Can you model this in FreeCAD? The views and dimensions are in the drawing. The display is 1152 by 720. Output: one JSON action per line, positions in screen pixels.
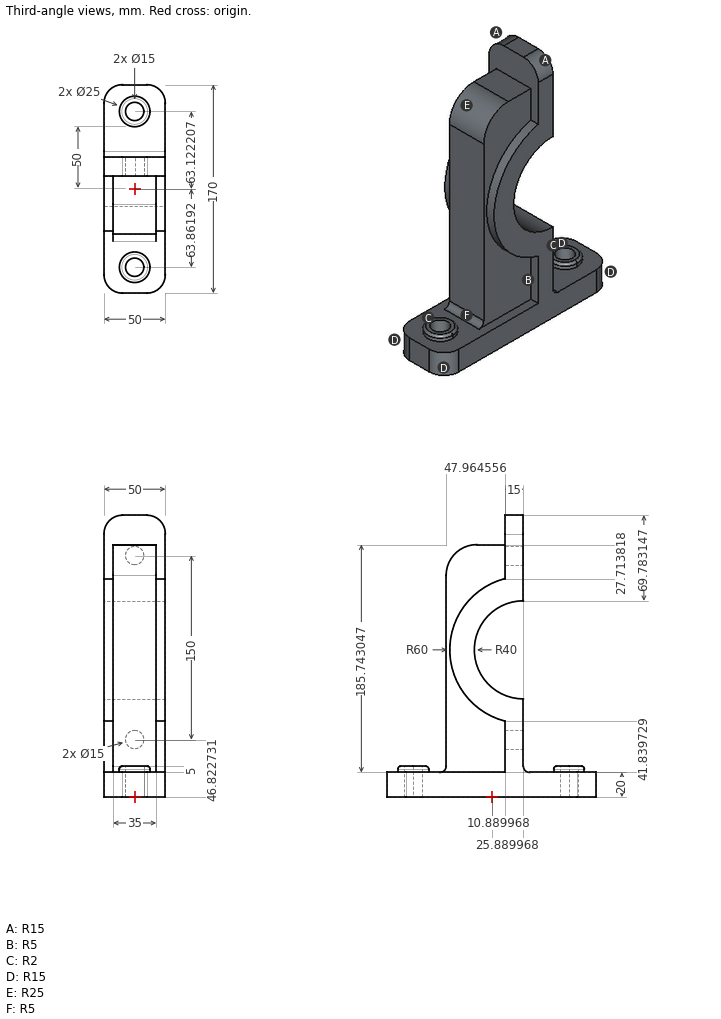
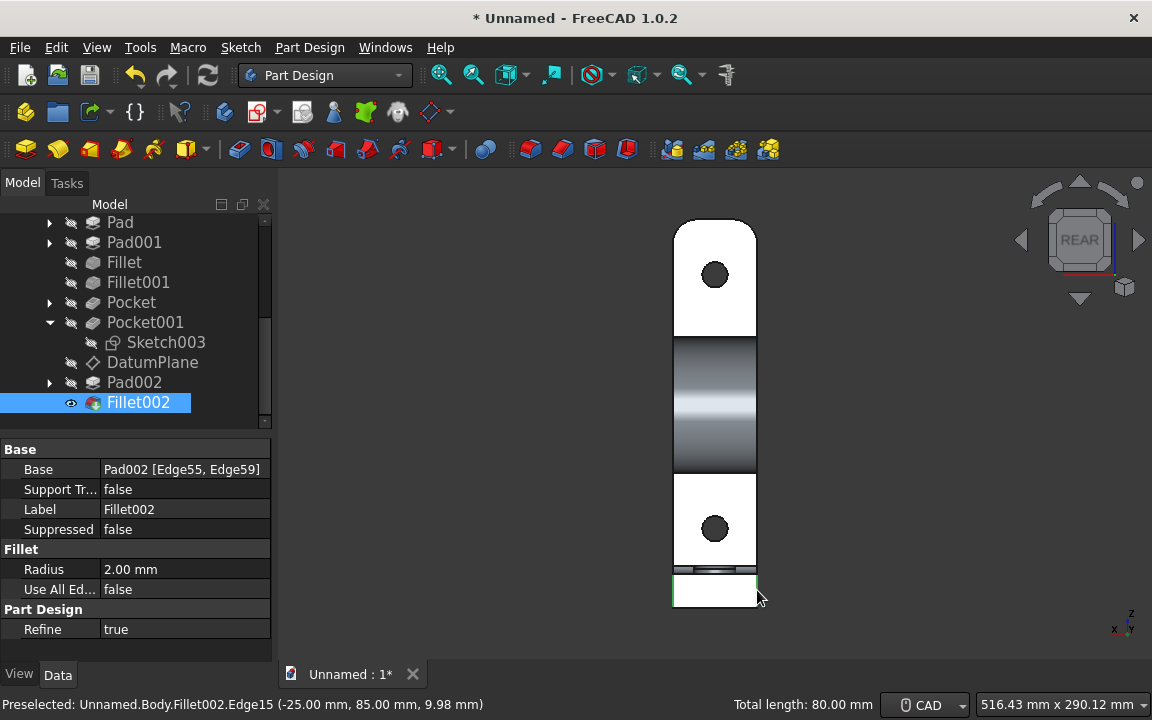
{"action": "left_click", "coordinate": [532, 150]}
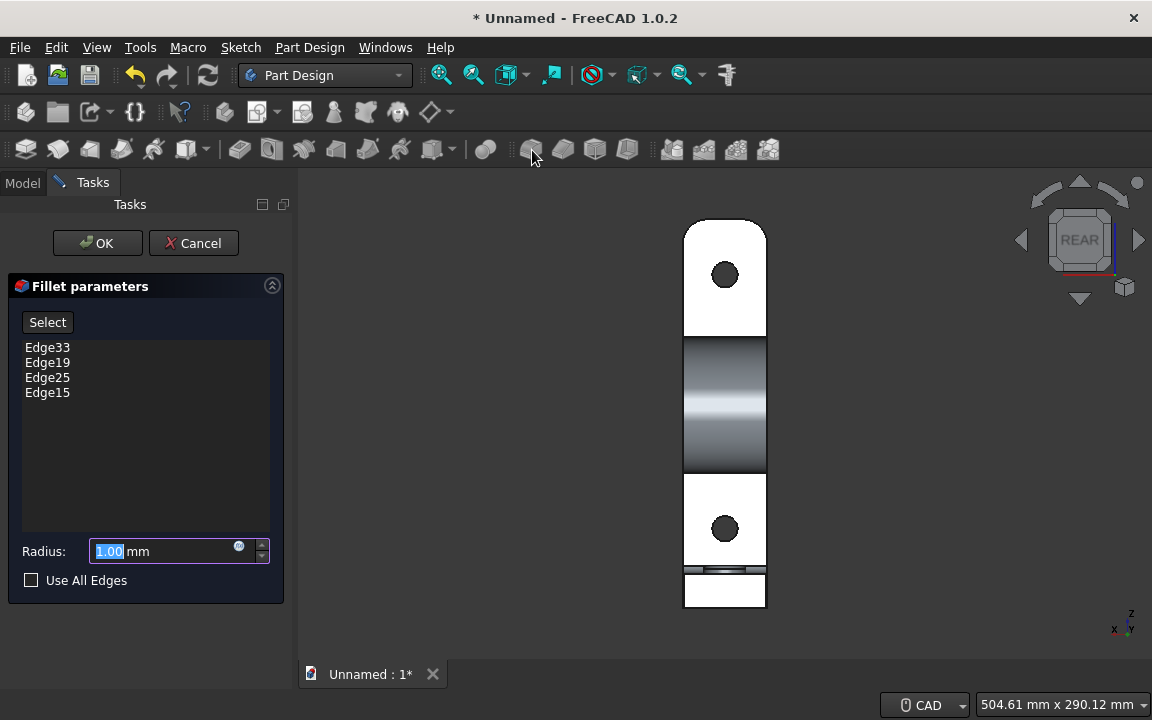
{"action": "type", "text": "15"}
{"action": "key", "text": "Tab"}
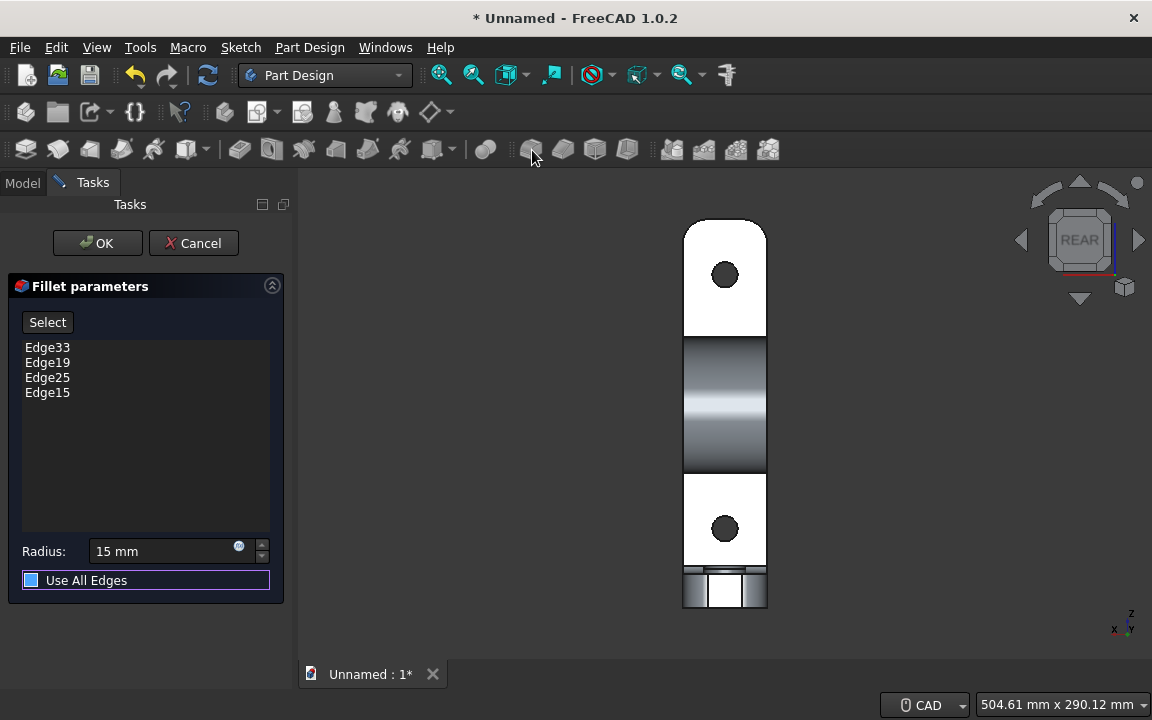
{"action": "left_click", "coordinate": [98, 243]}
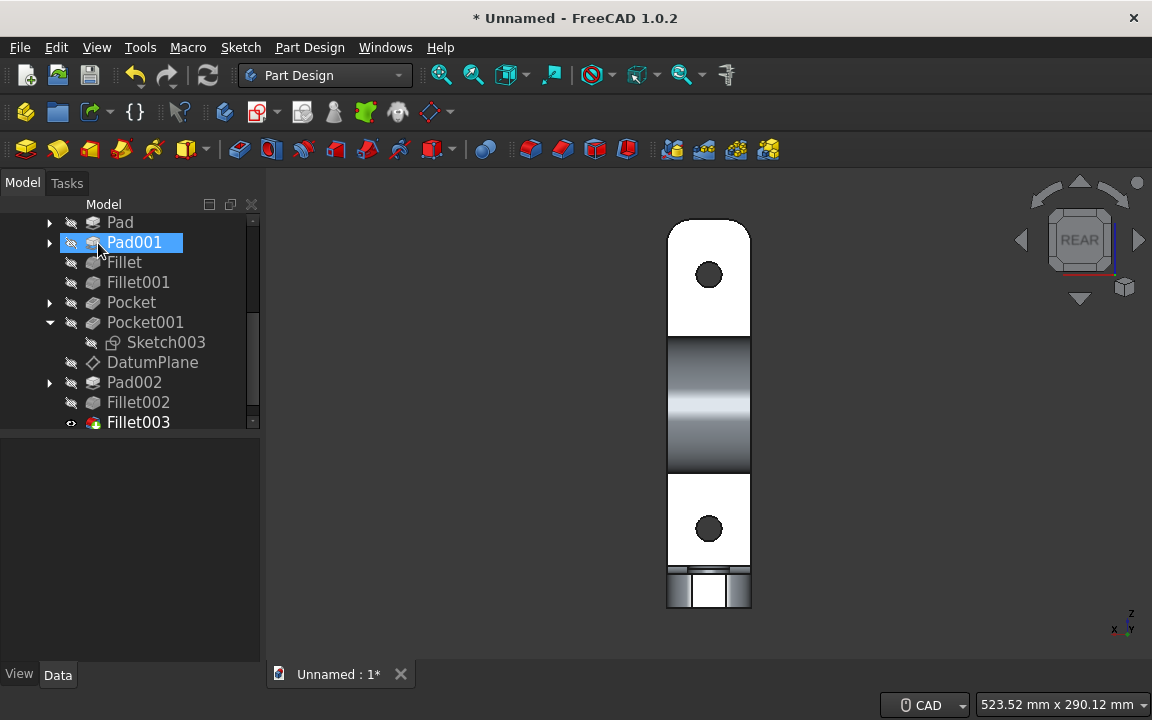
{"action": "left_click", "coordinate": [258, 112]}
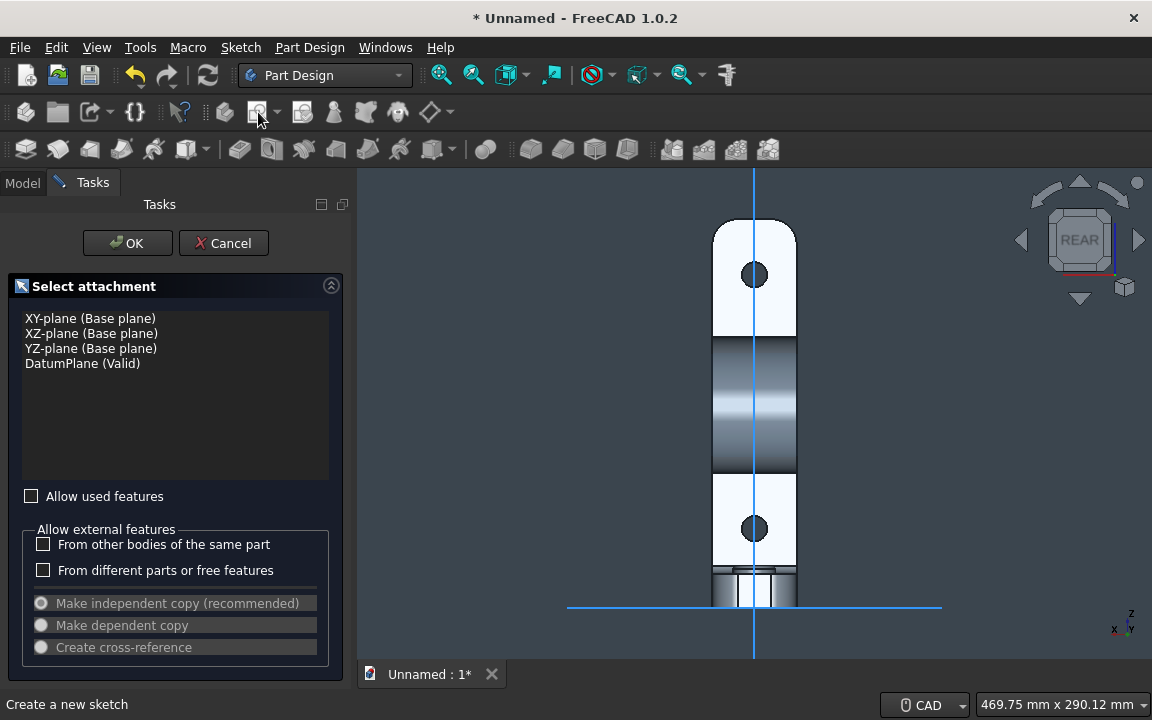
{"action": "left_click", "coordinate": [82, 348]}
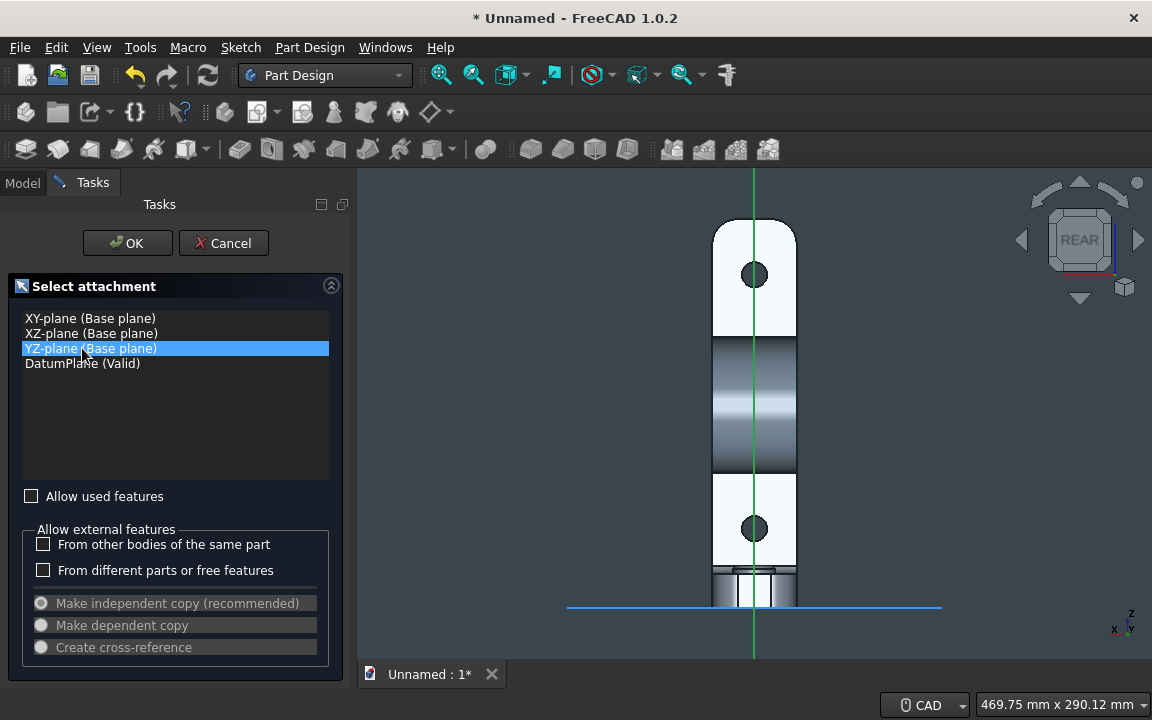
{"action": "left_click", "coordinate": [128, 243]}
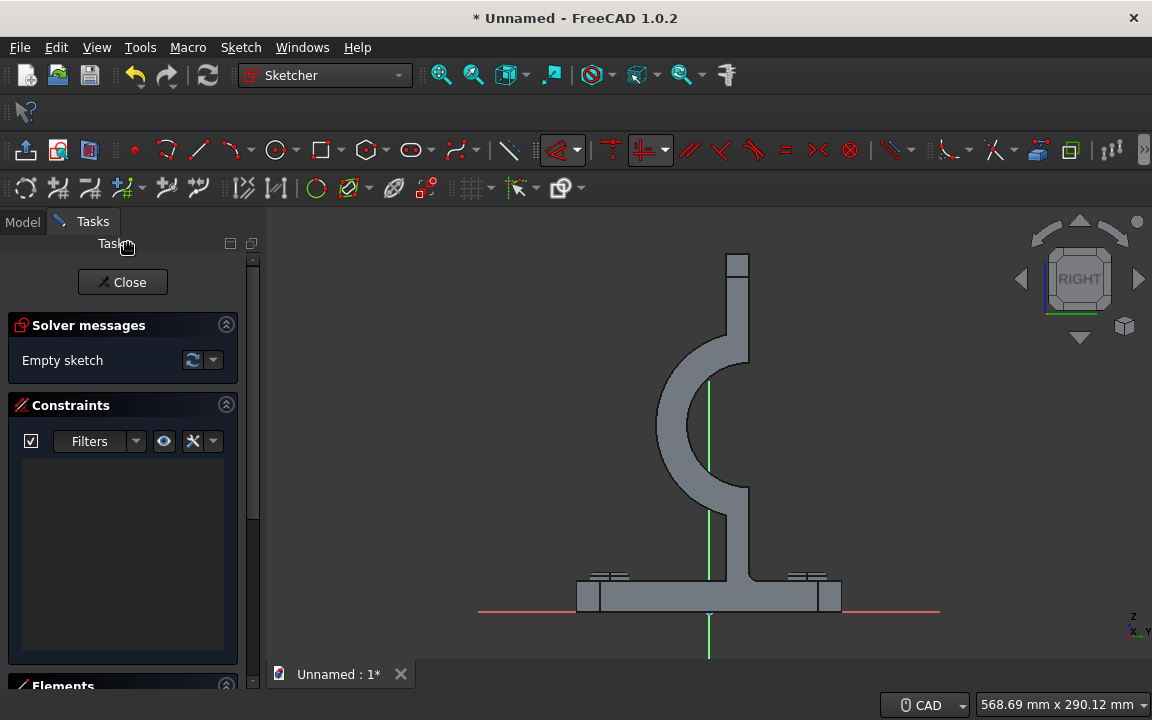
{"action": "key", "text": "q s"}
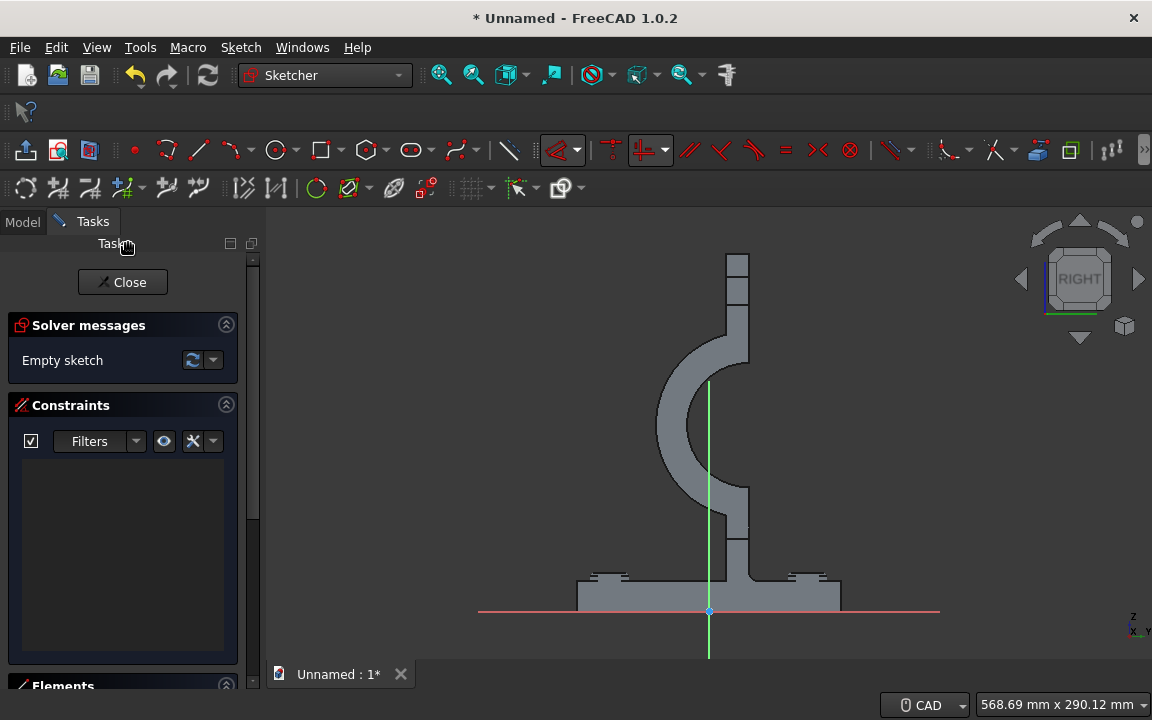
{"action": "scroll", "coordinate": [423, 349], "scroll_direction": "down", "scroll_amount": 1}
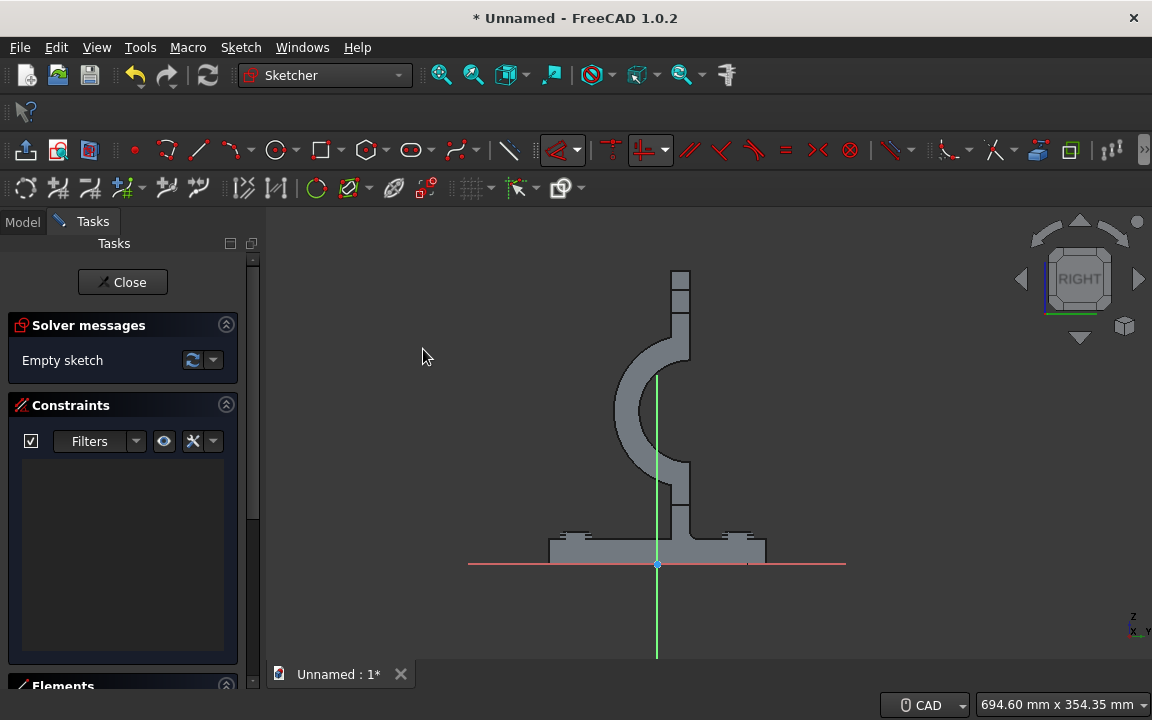
{"action": "key", "text": "g m"}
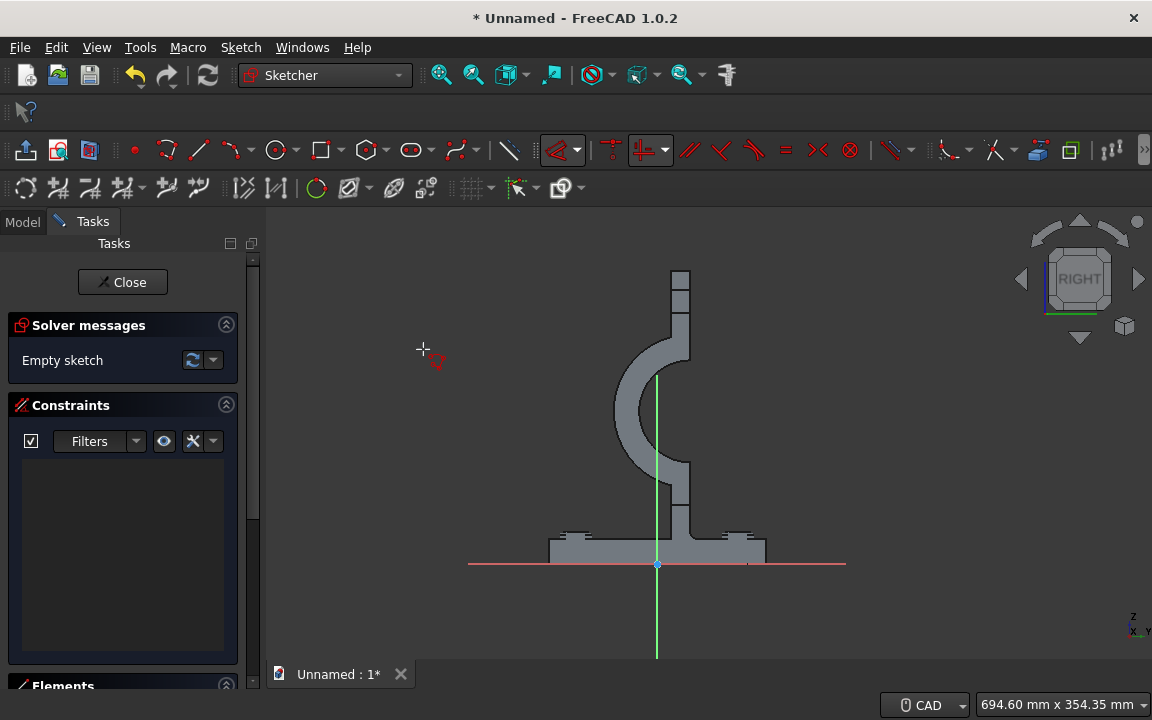
{"action": "left_click", "coordinate": [671, 337]}
{"action": "left_click", "coordinate": [671, 302]}
{"action": "left_click", "coordinate": [610, 302]}
{"action": "left_click", "coordinate": [610, 539]}
{"action": "left_click", "coordinate": [671, 539]}
{"action": "left_click", "coordinate": [671, 485]}
{"action": "right_click", "coordinate": [671, 485]}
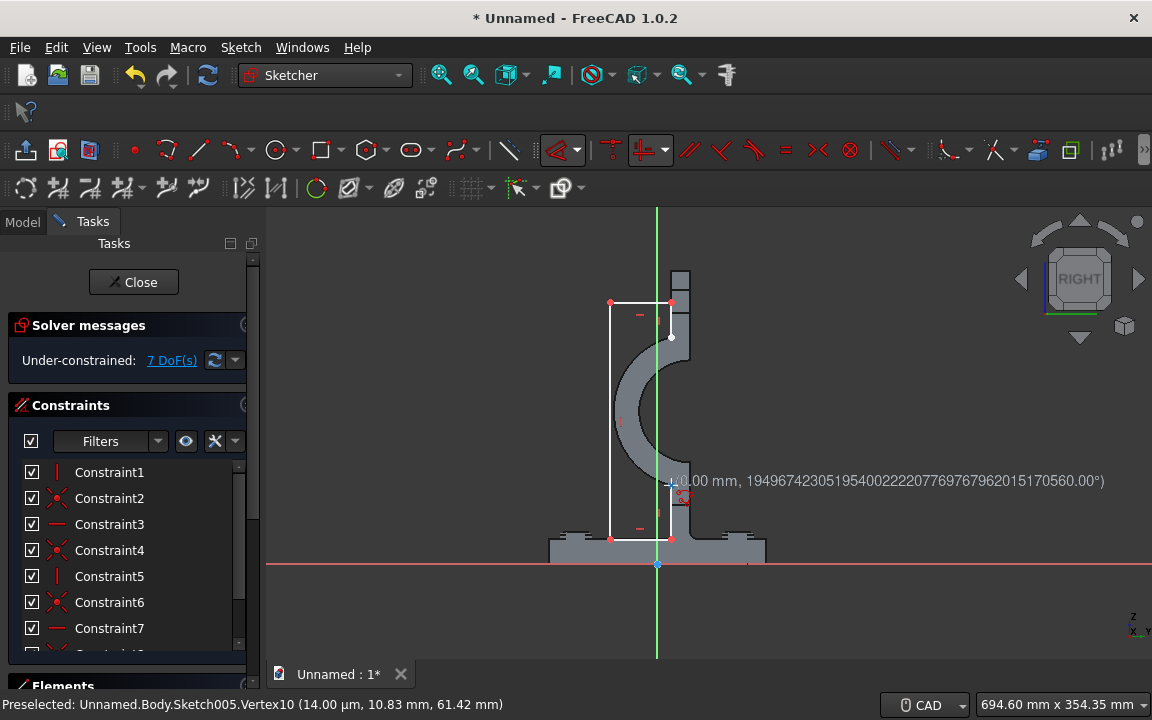
{"action": "key", "text": "g 3 a"}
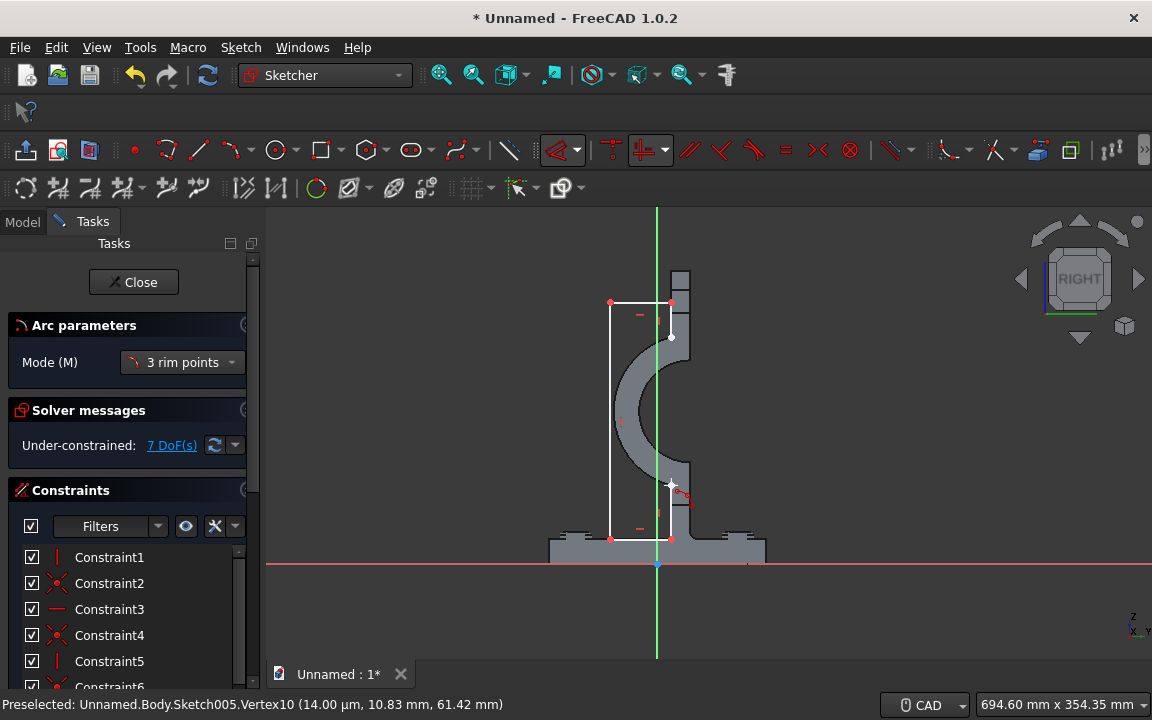
{"action": "left_click", "coordinate": [671, 486]}
{"action": "left_click", "coordinate": [671, 338]}
{"action": "left_click", "coordinate": [624, 373]}
{"action": "key", "text": "Escape"}